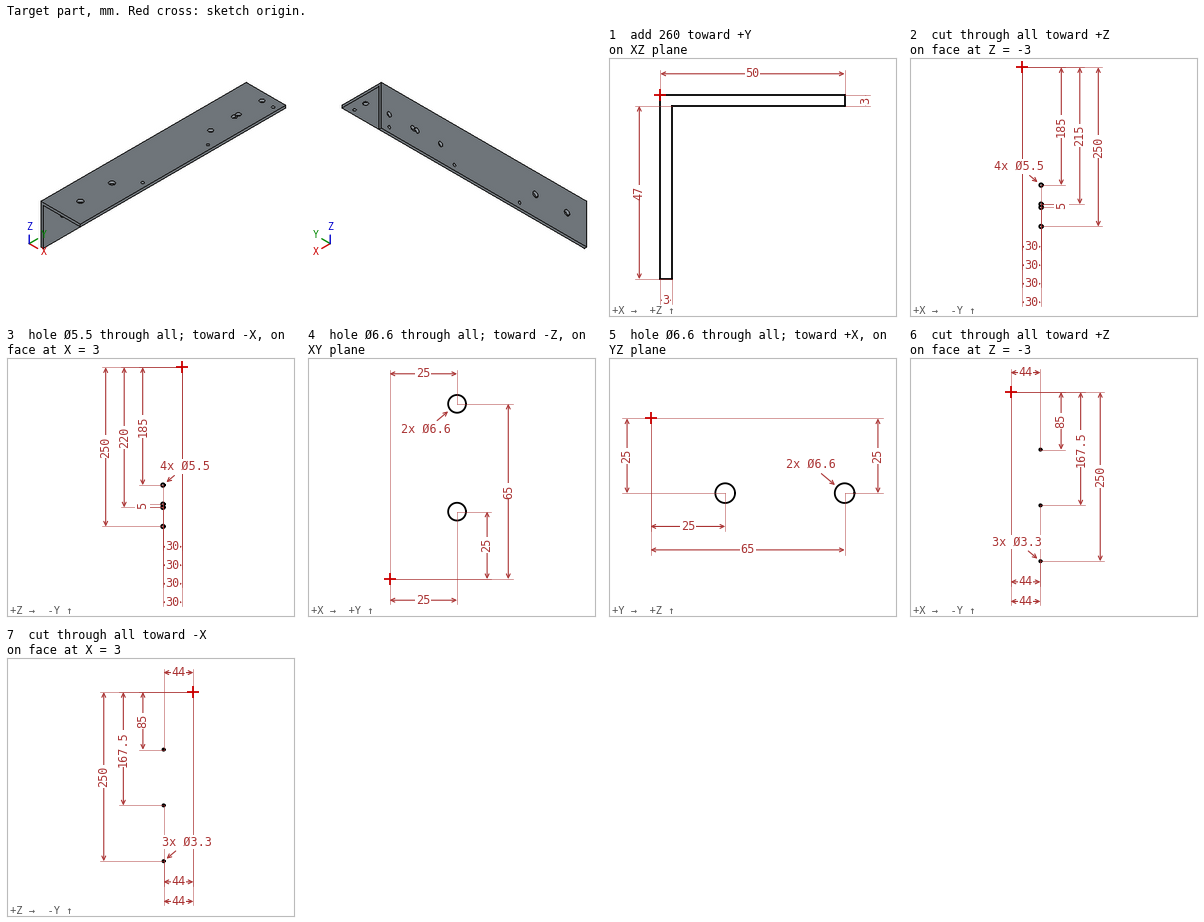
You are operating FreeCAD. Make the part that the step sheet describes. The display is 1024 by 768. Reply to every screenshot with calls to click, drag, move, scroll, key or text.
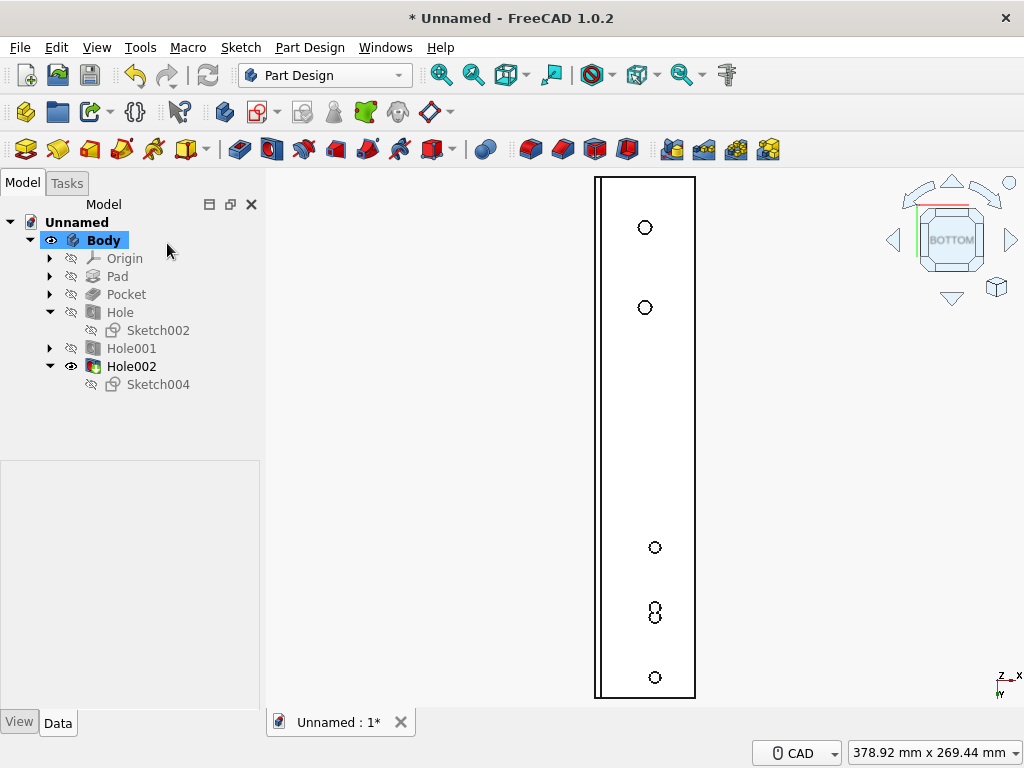
click(648, 437)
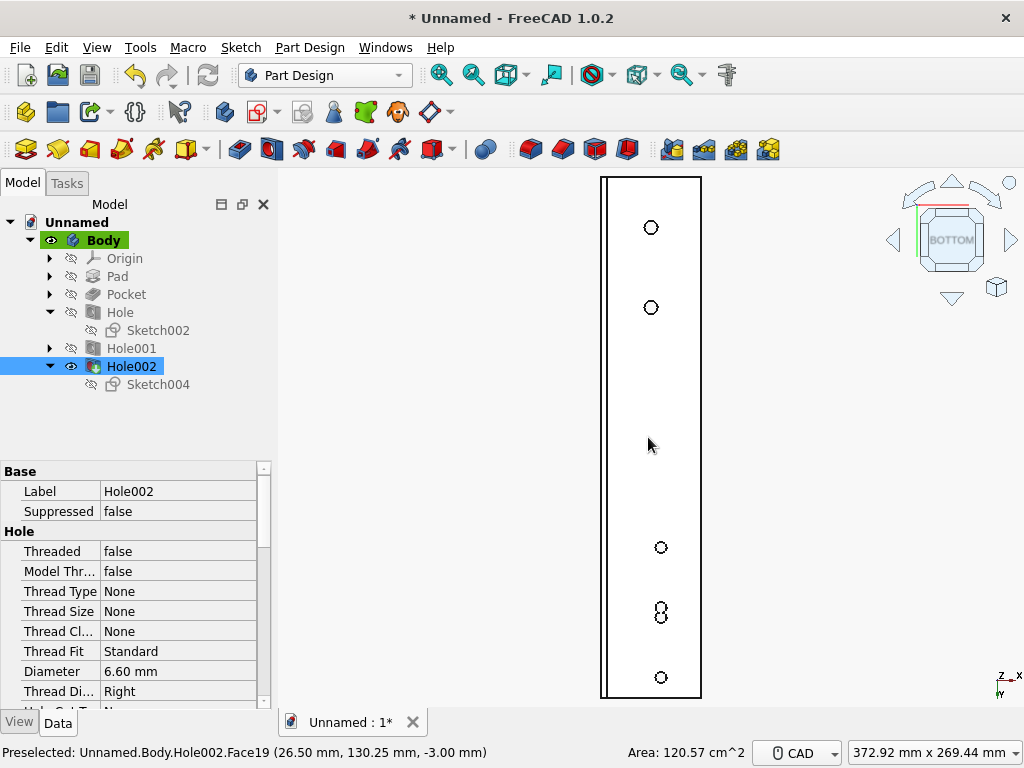
click(258, 112)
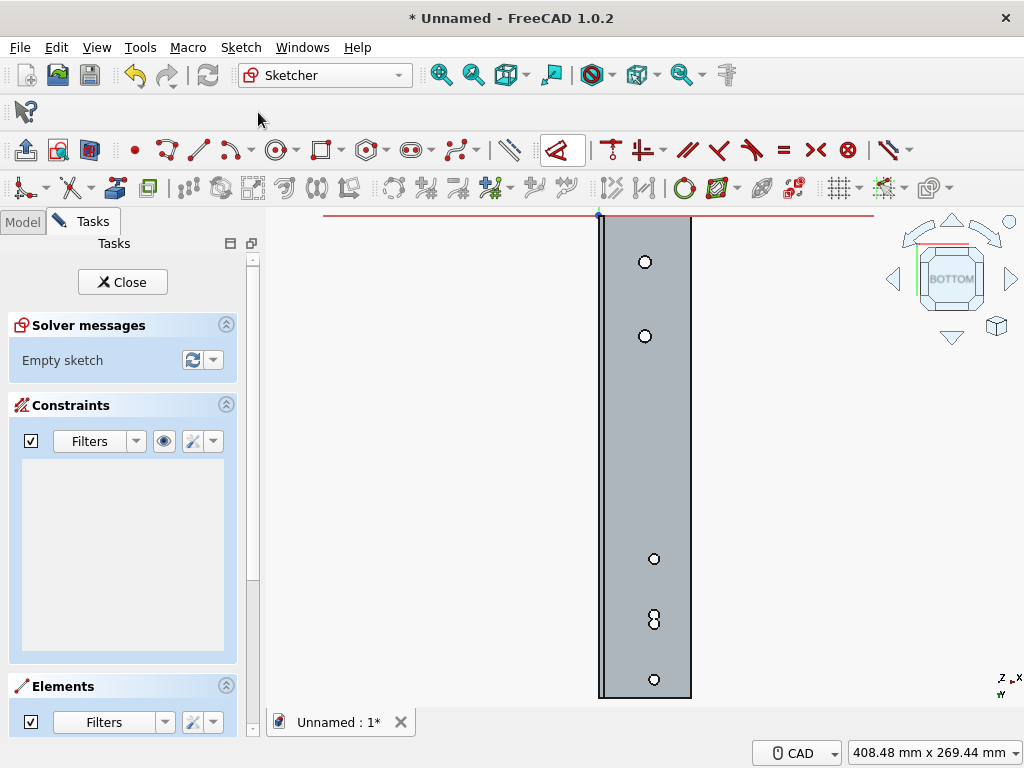
click(90, 150)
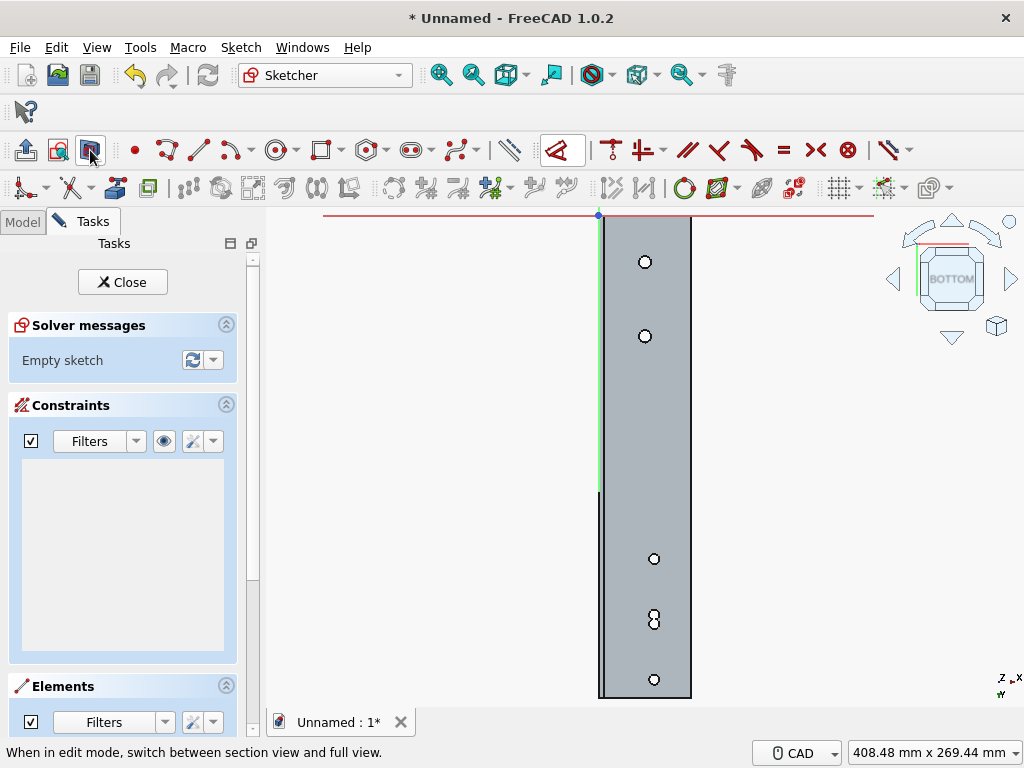
scroll(445, 473, down, 2)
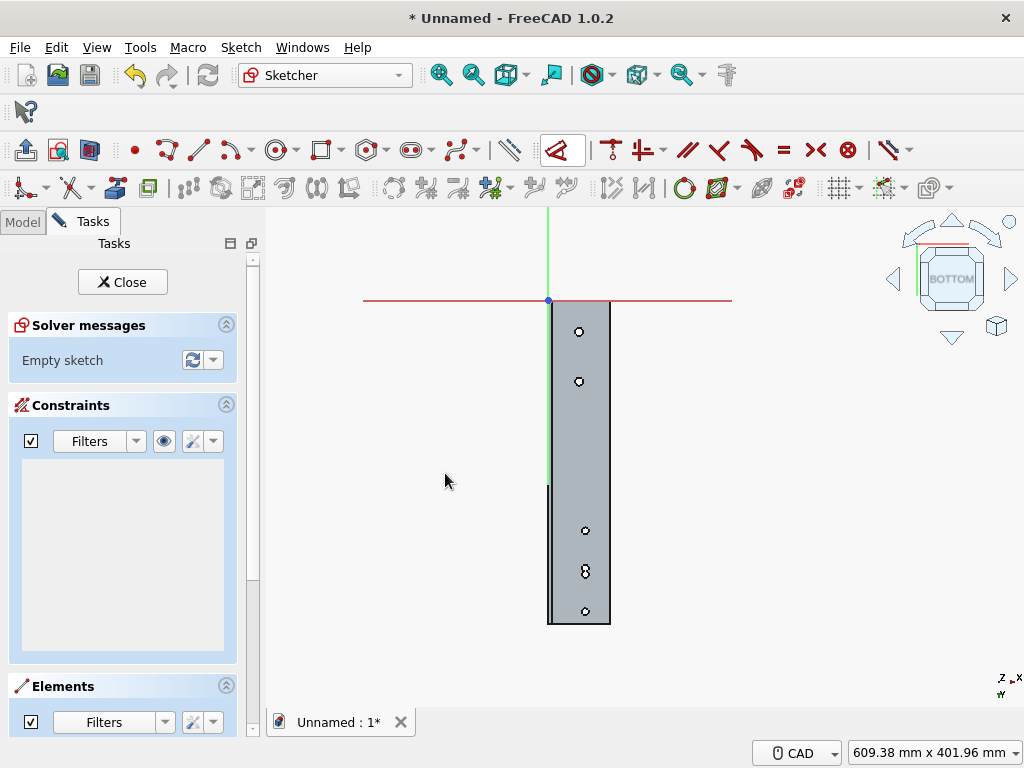
click(276, 150)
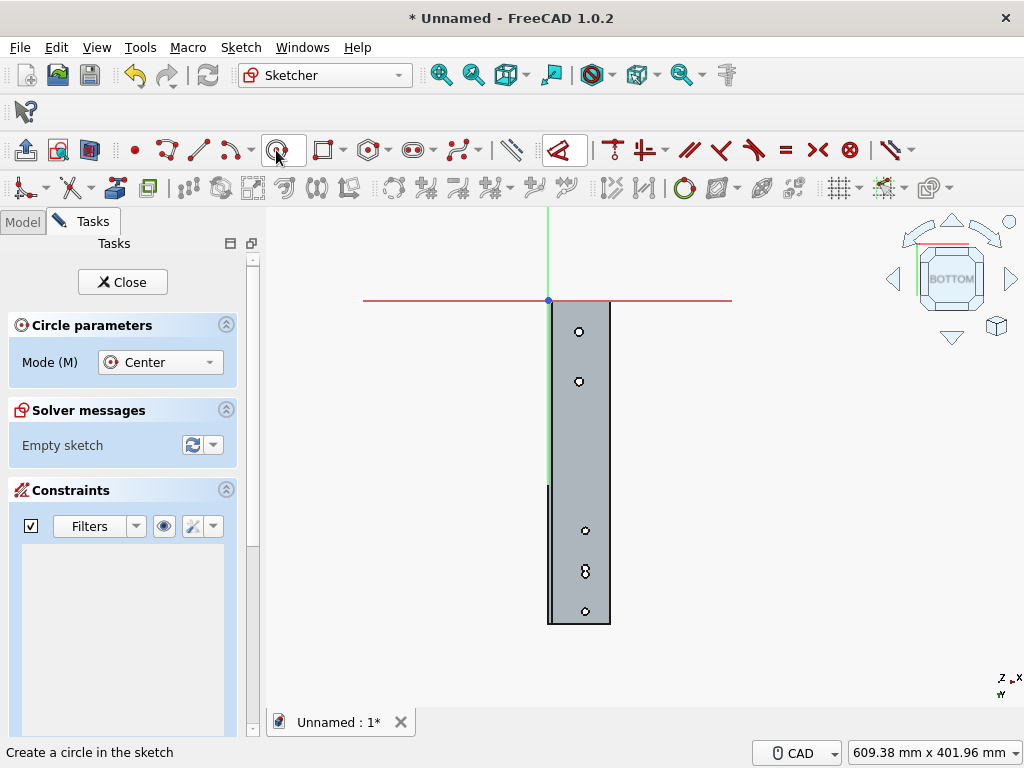
scroll(603, 612, up, 13)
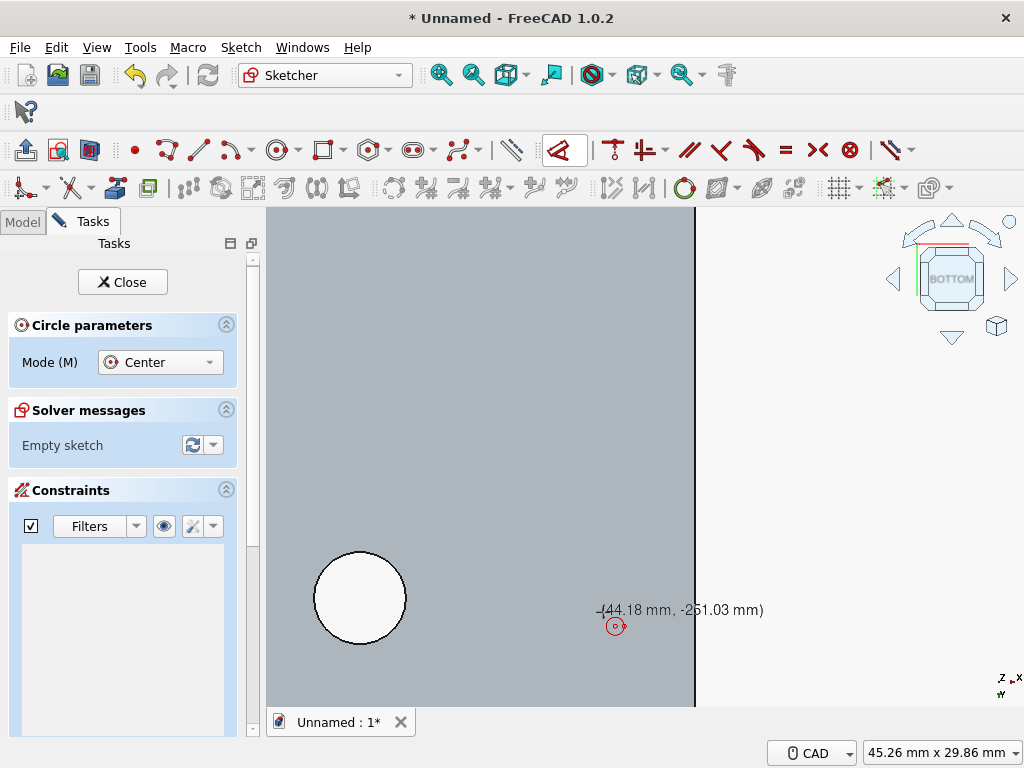
scroll(604, 613, down, 13)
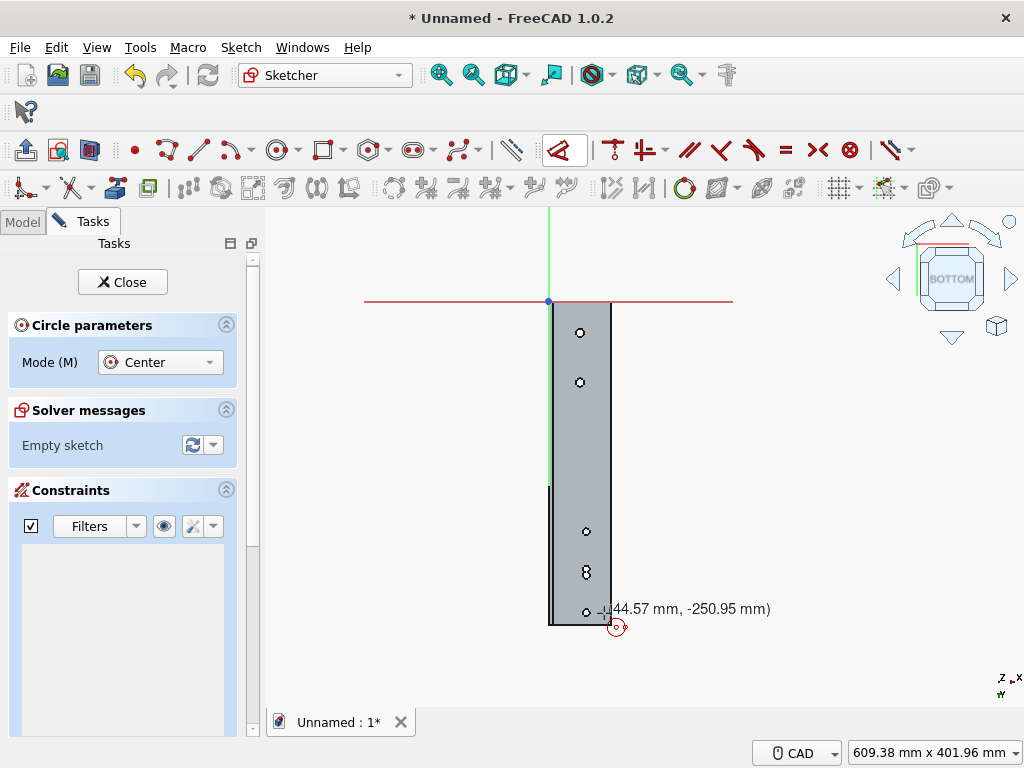
click(604, 613)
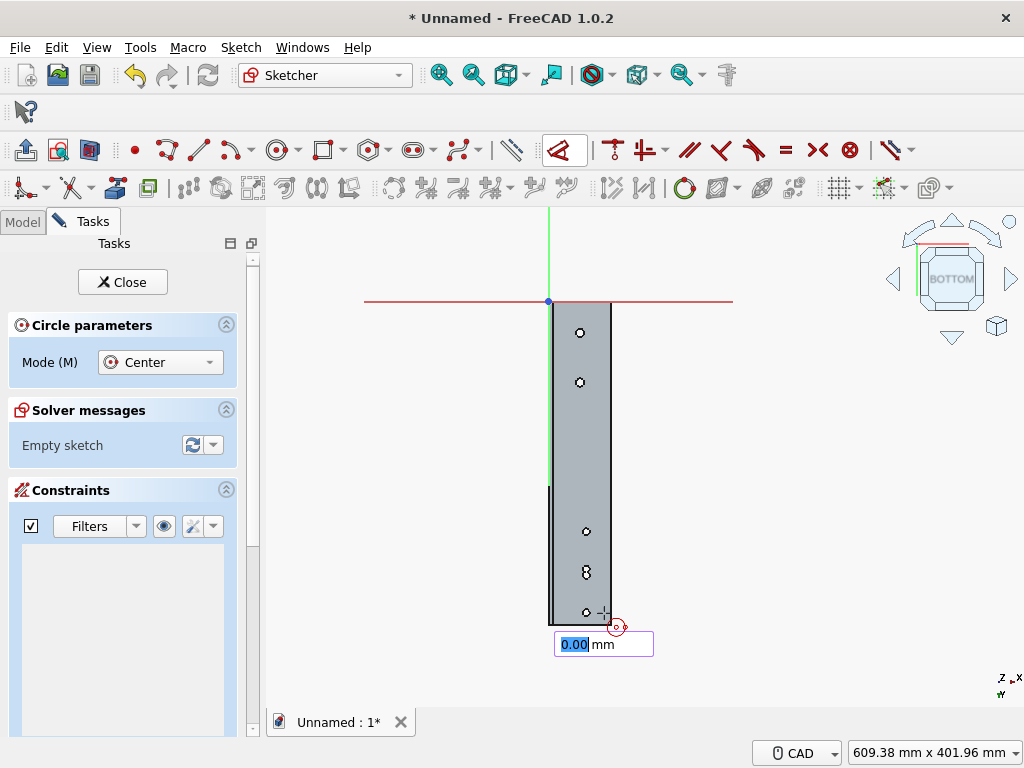
scroll(605, 611, up, 11)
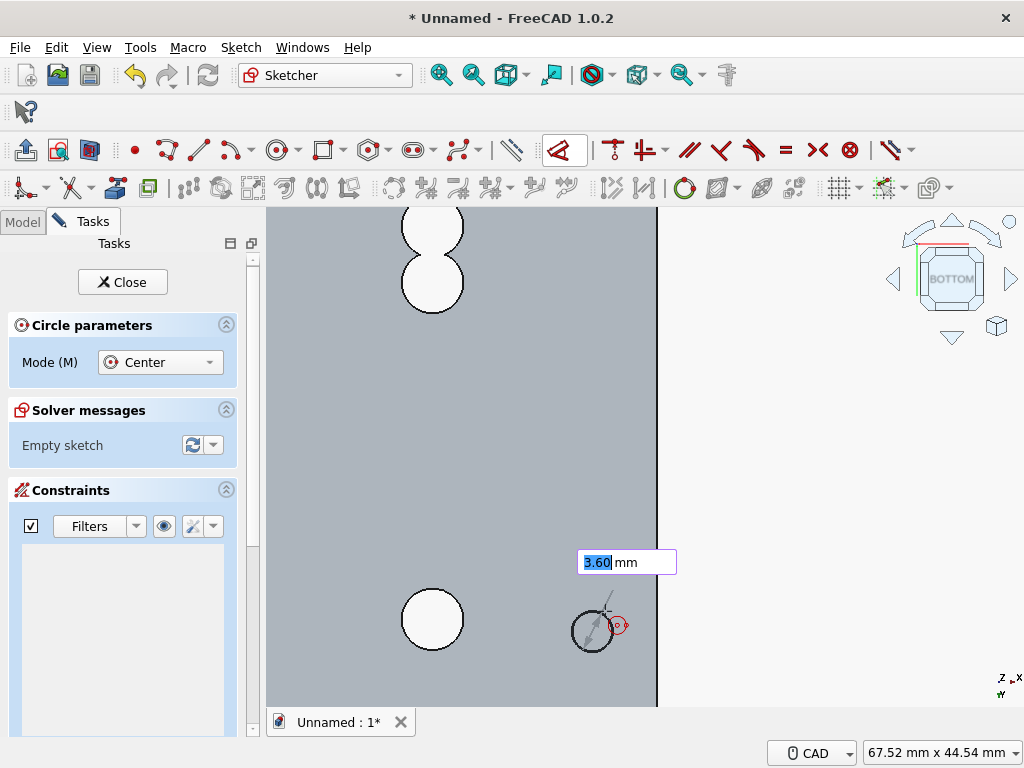
click(603, 606)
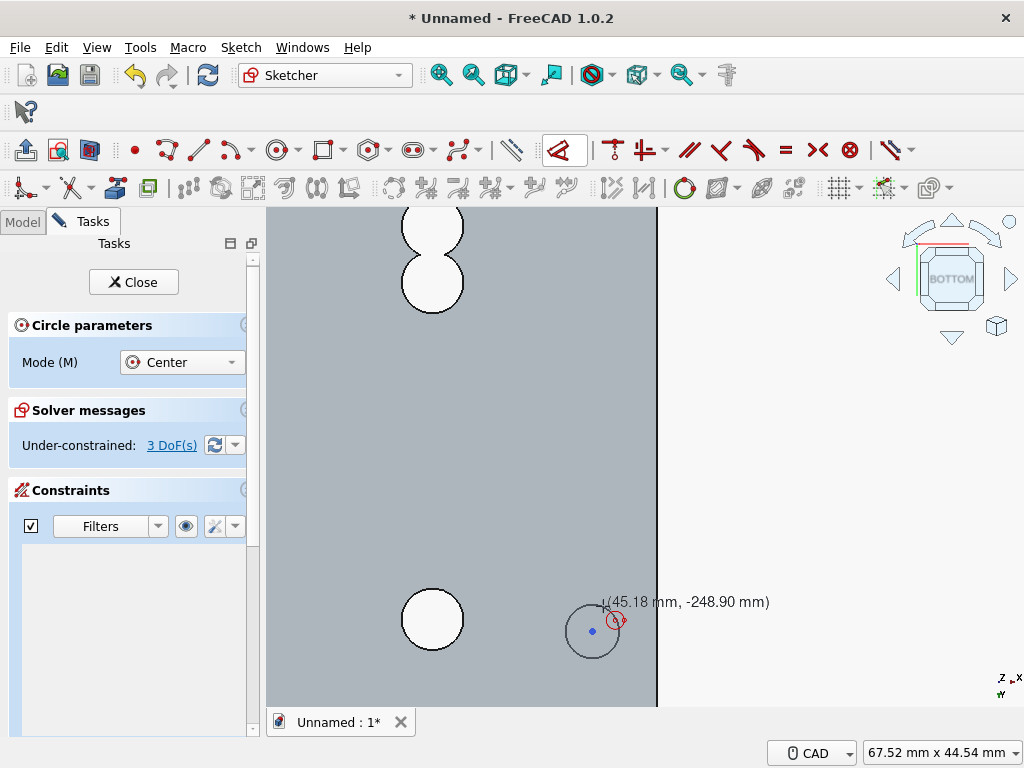
scroll(604, 610, down, 11)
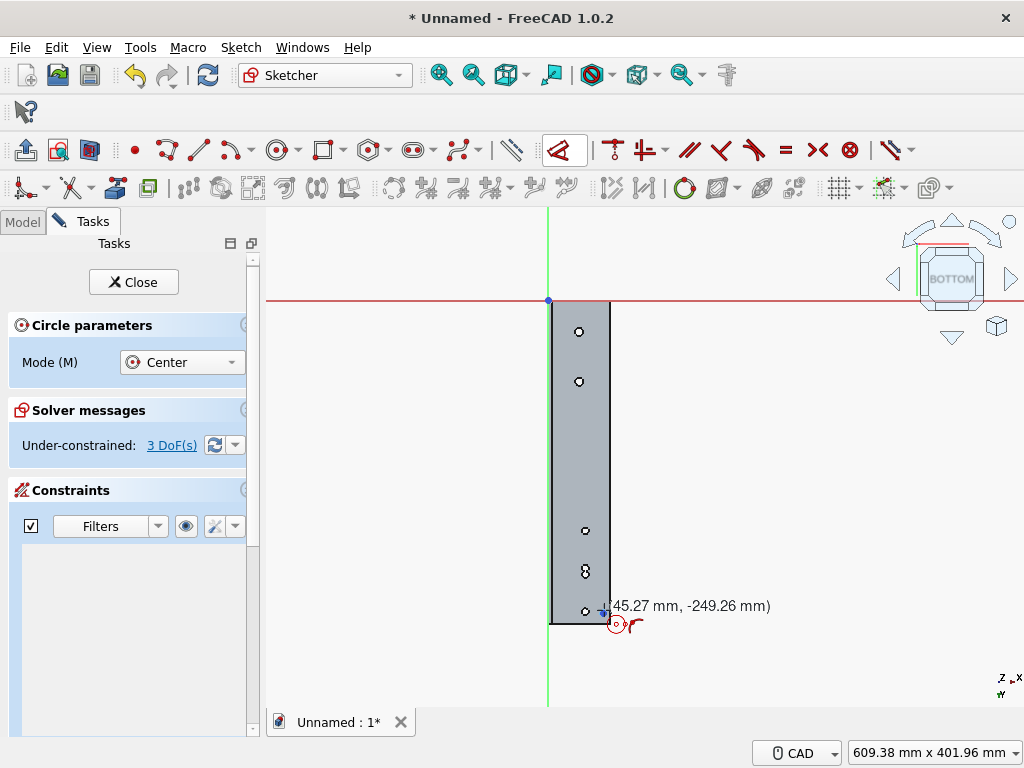
scroll(603, 509, up, 13)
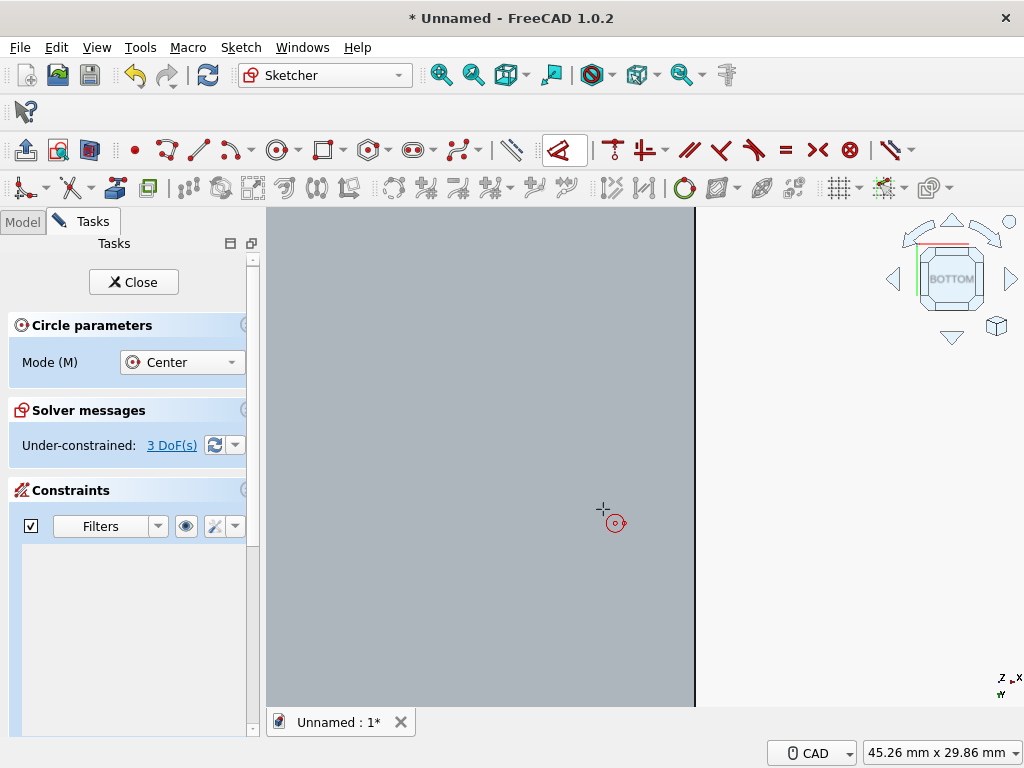
scroll(603, 509, down, 13)